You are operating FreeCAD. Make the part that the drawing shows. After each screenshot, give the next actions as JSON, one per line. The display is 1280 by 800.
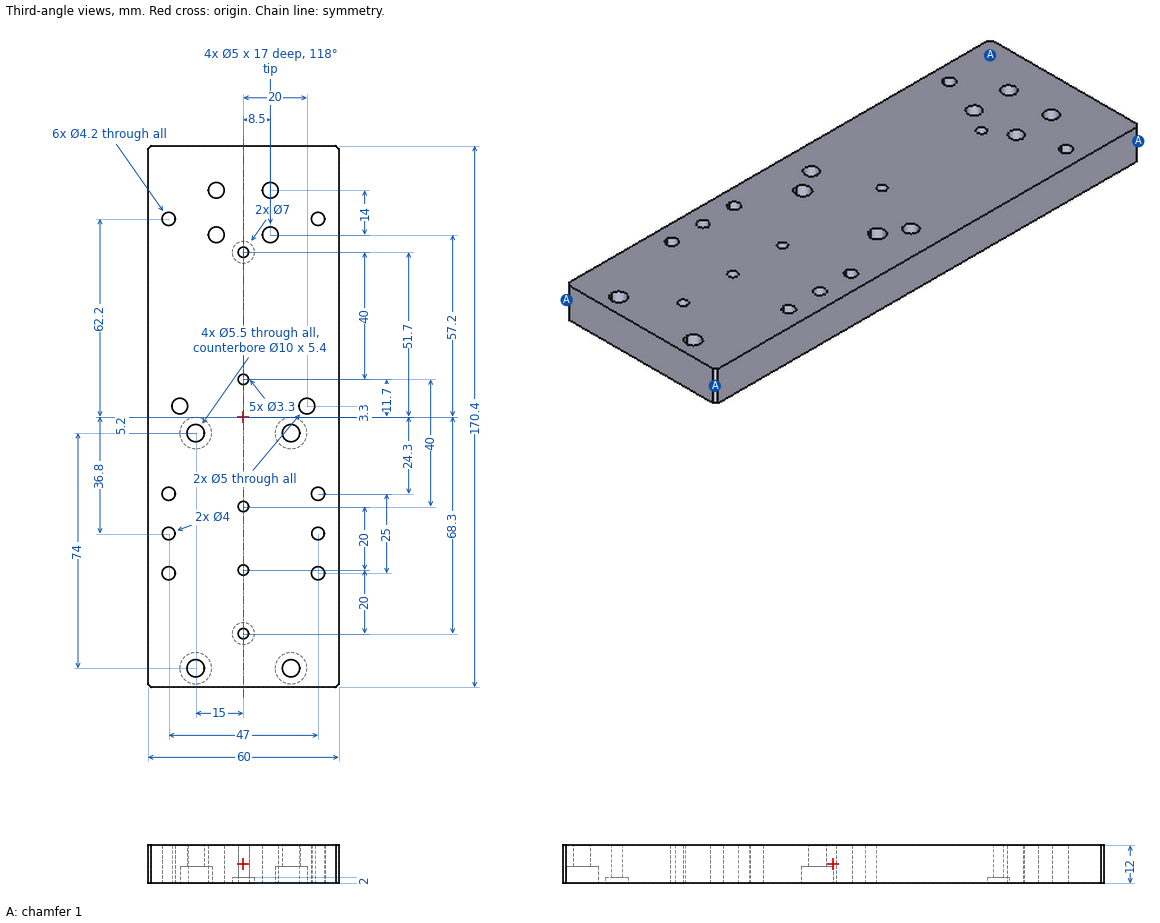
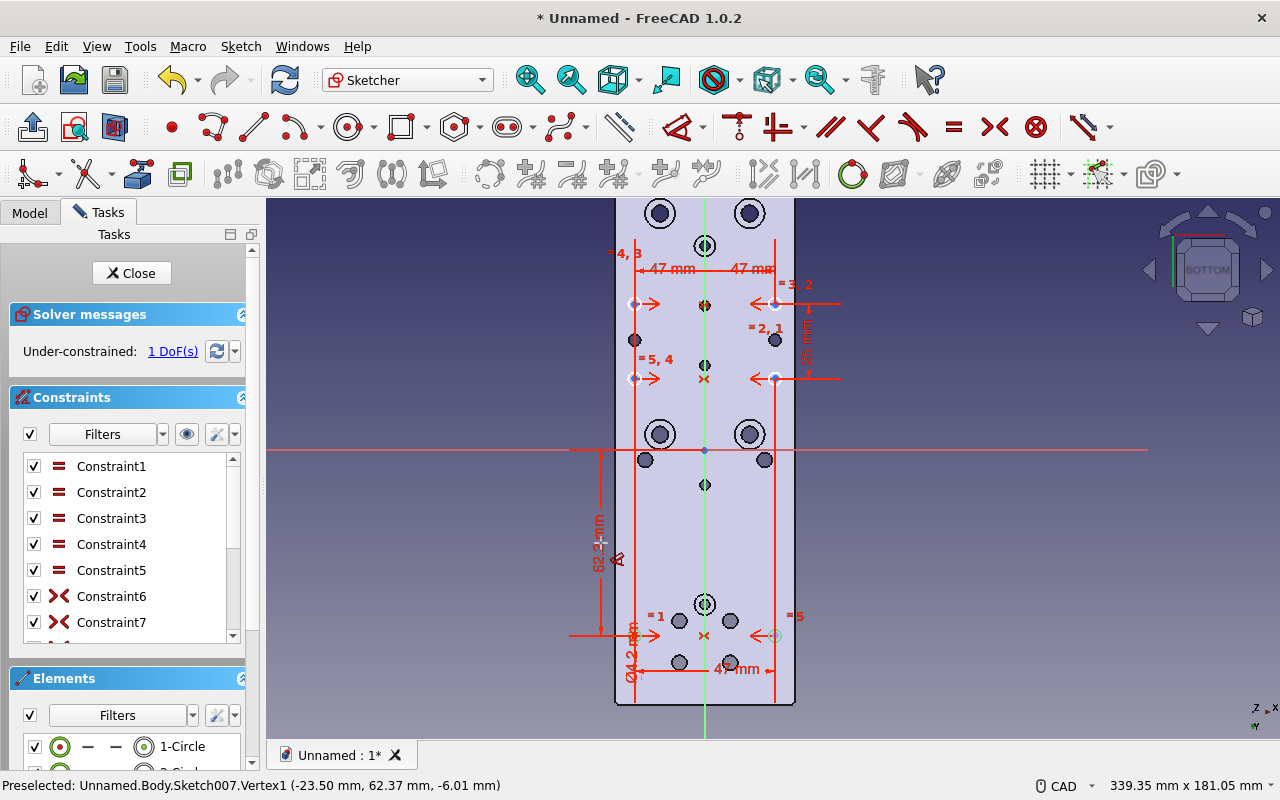
{"action": "left_click", "coordinate": [775, 379]}
{"action": "left_click", "coordinate": [809, 414]}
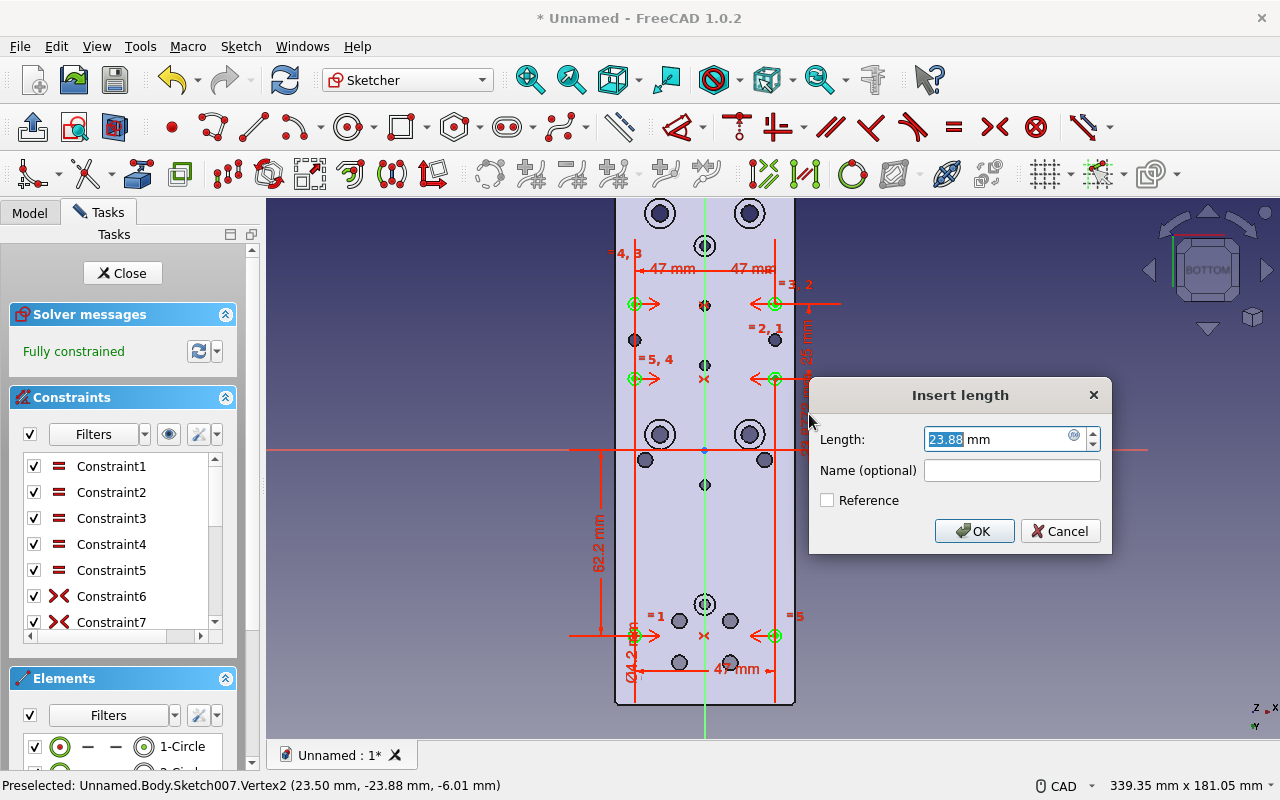
{"action": "type", "text": "24.3"}
{"action": "key", "text": "Return"}
{"action": "key", "text": "Escape"}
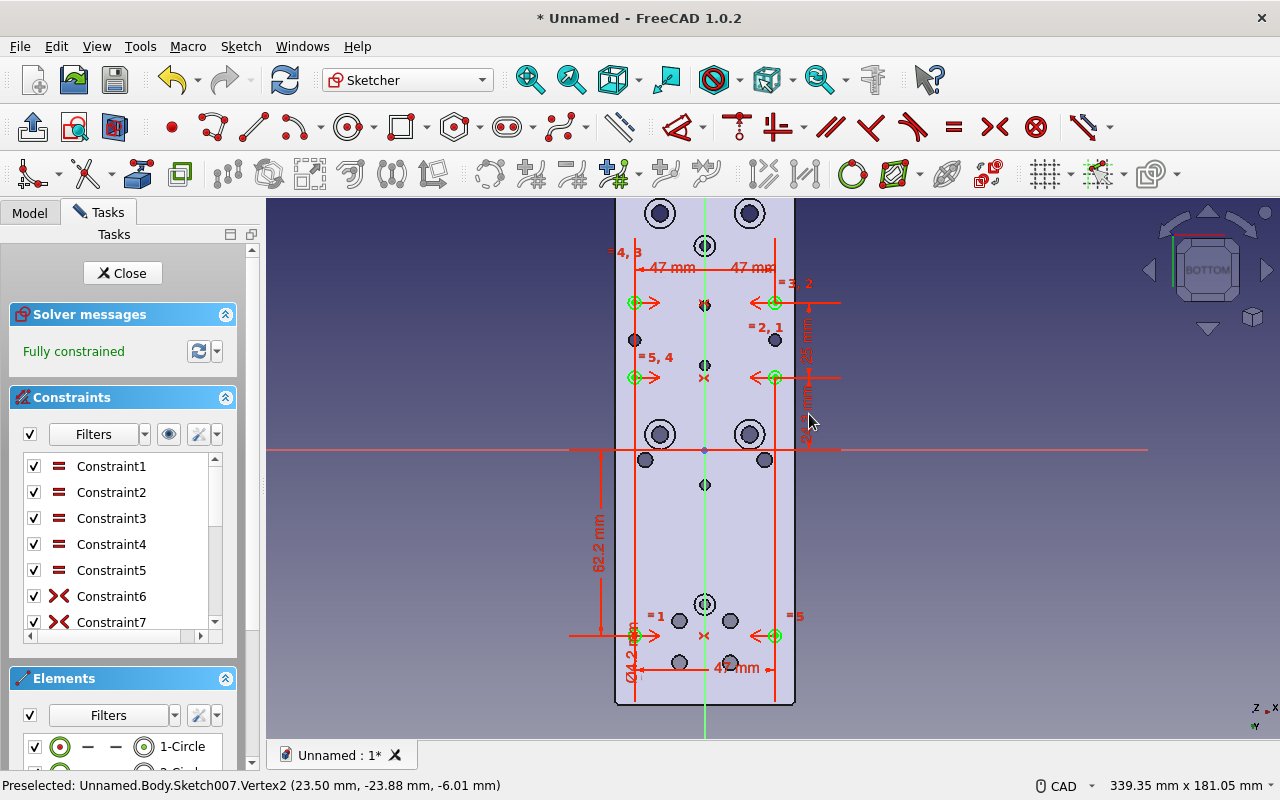
{"action": "left_click", "coordinate": [123, 273]}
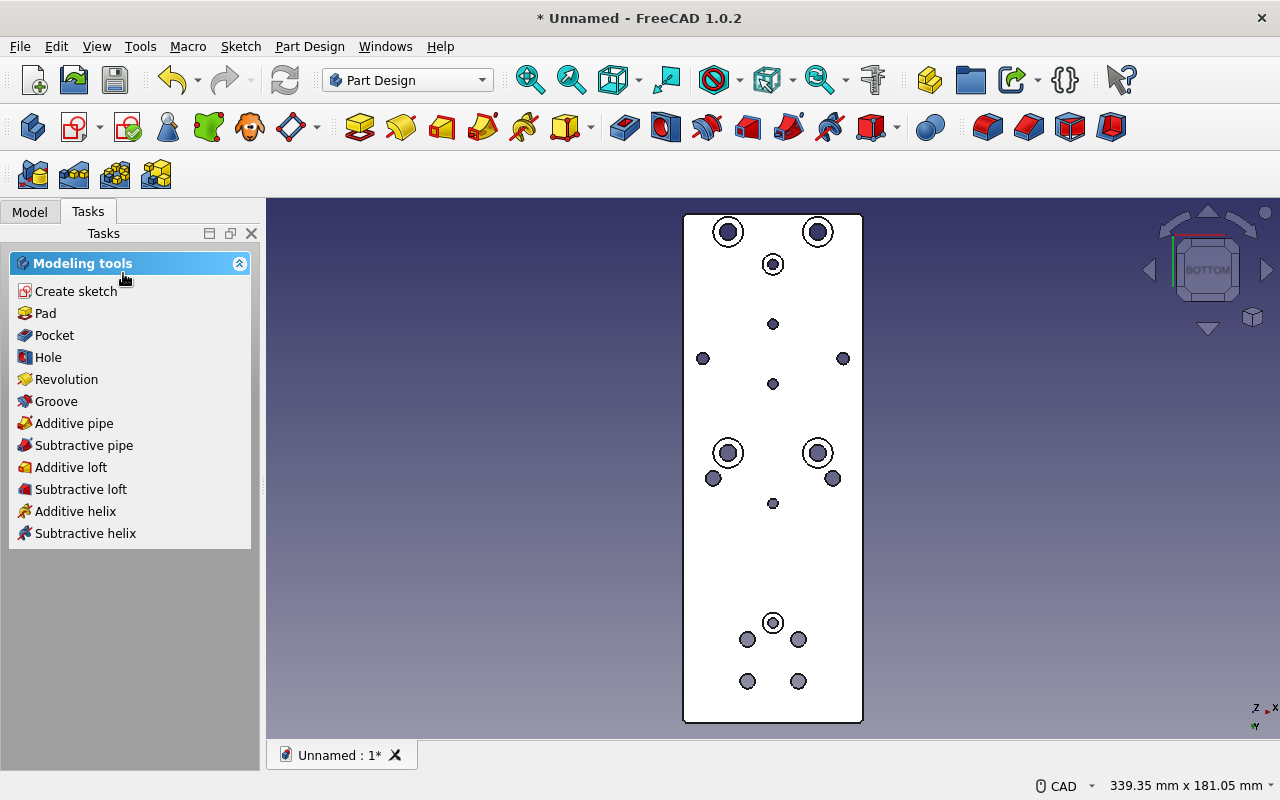
{"action": "left_click", "coordinate": [666, 128]}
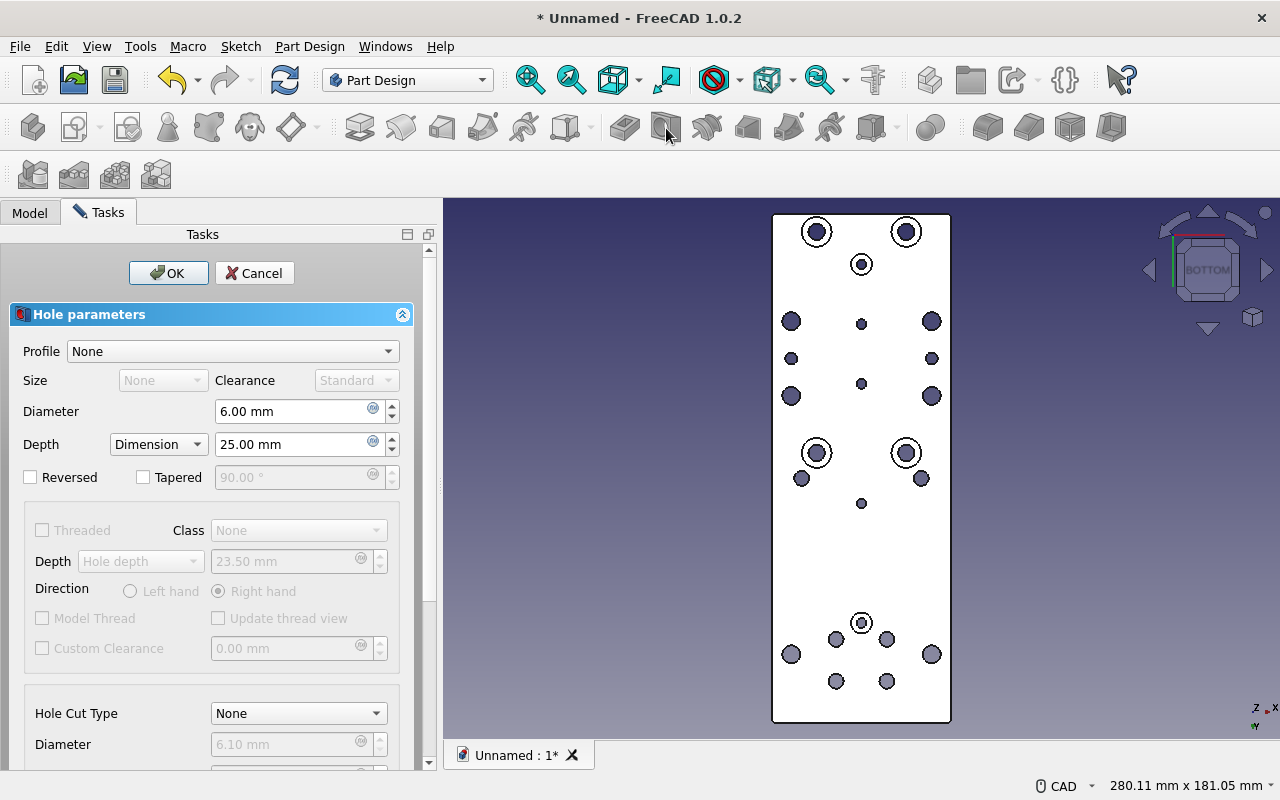
{"action": "triple_click", "coordinate": [300, 412]}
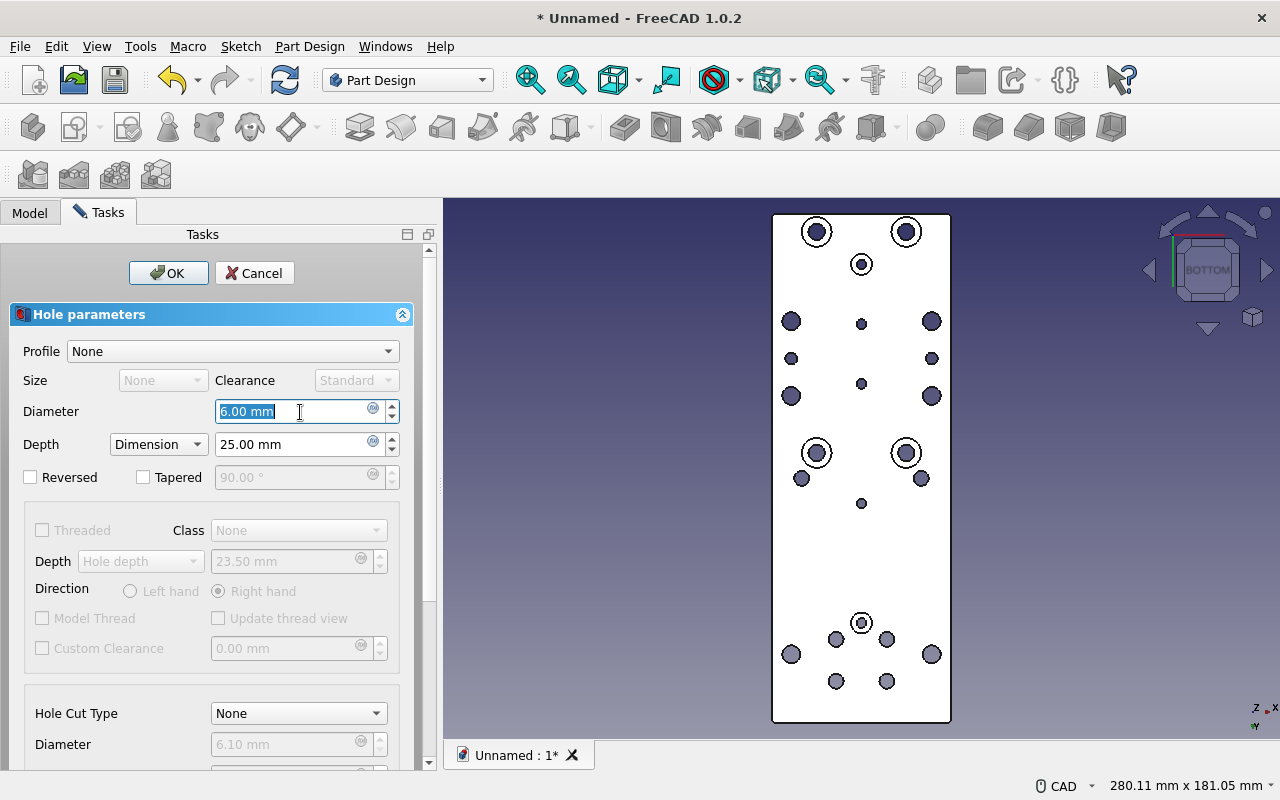
{"action": "type", "text": "4.2"}
{"action": "key", "text": "Tab"}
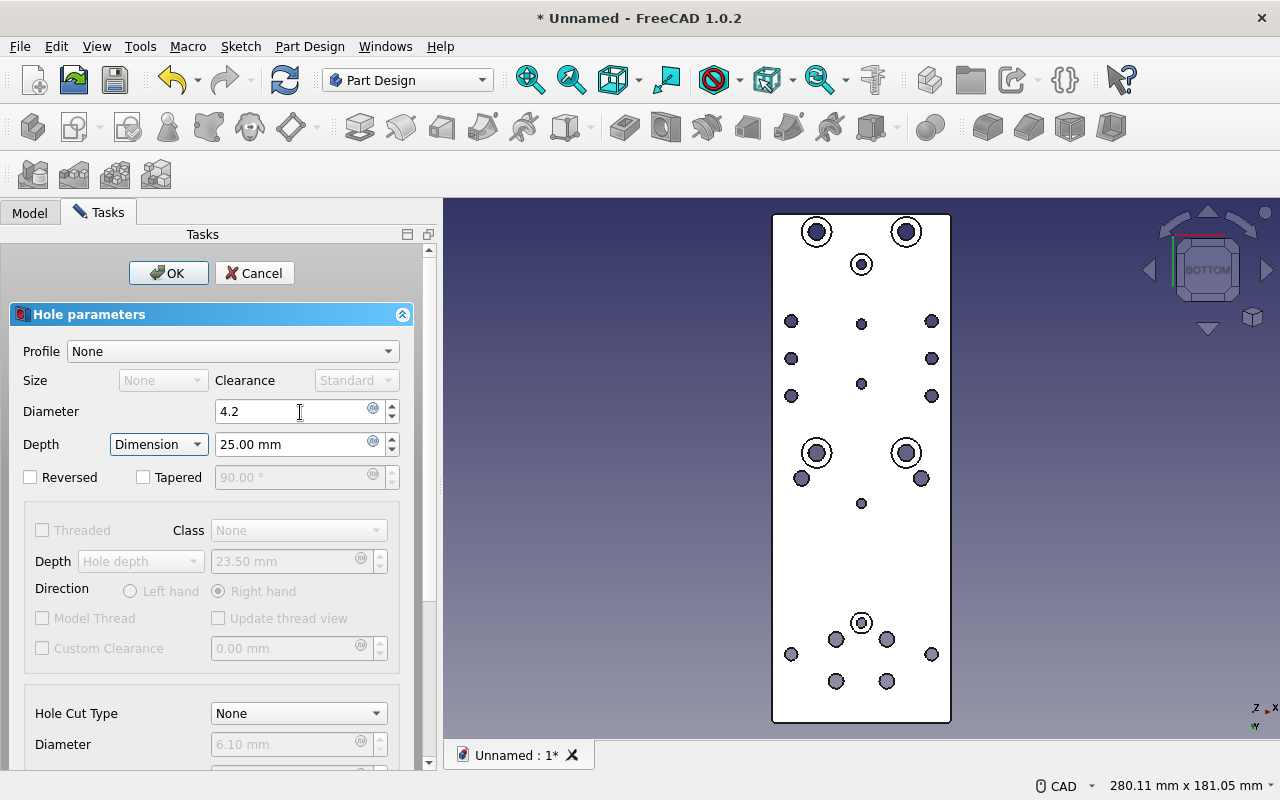
{"action": "left_click", "coordinate": [160, 444]}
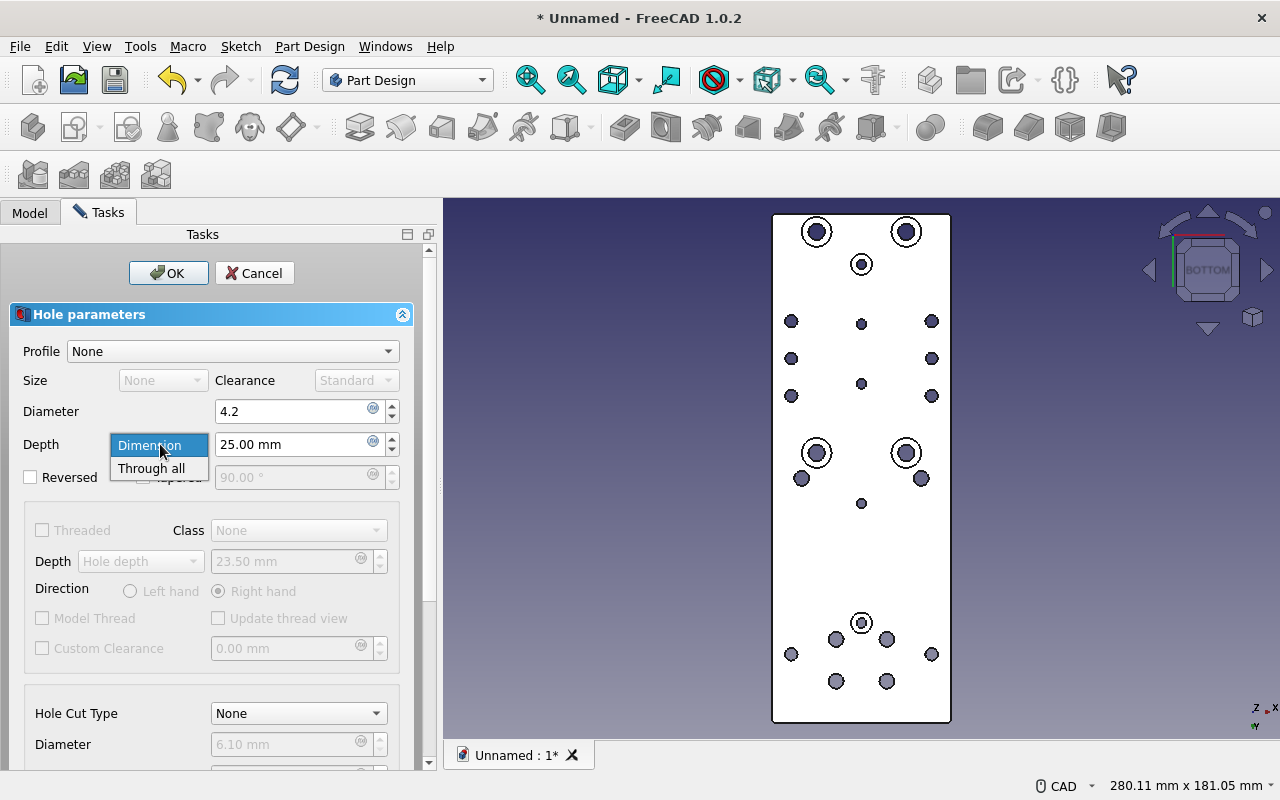
{"action": "left_click", "coordinate": [158, 468]}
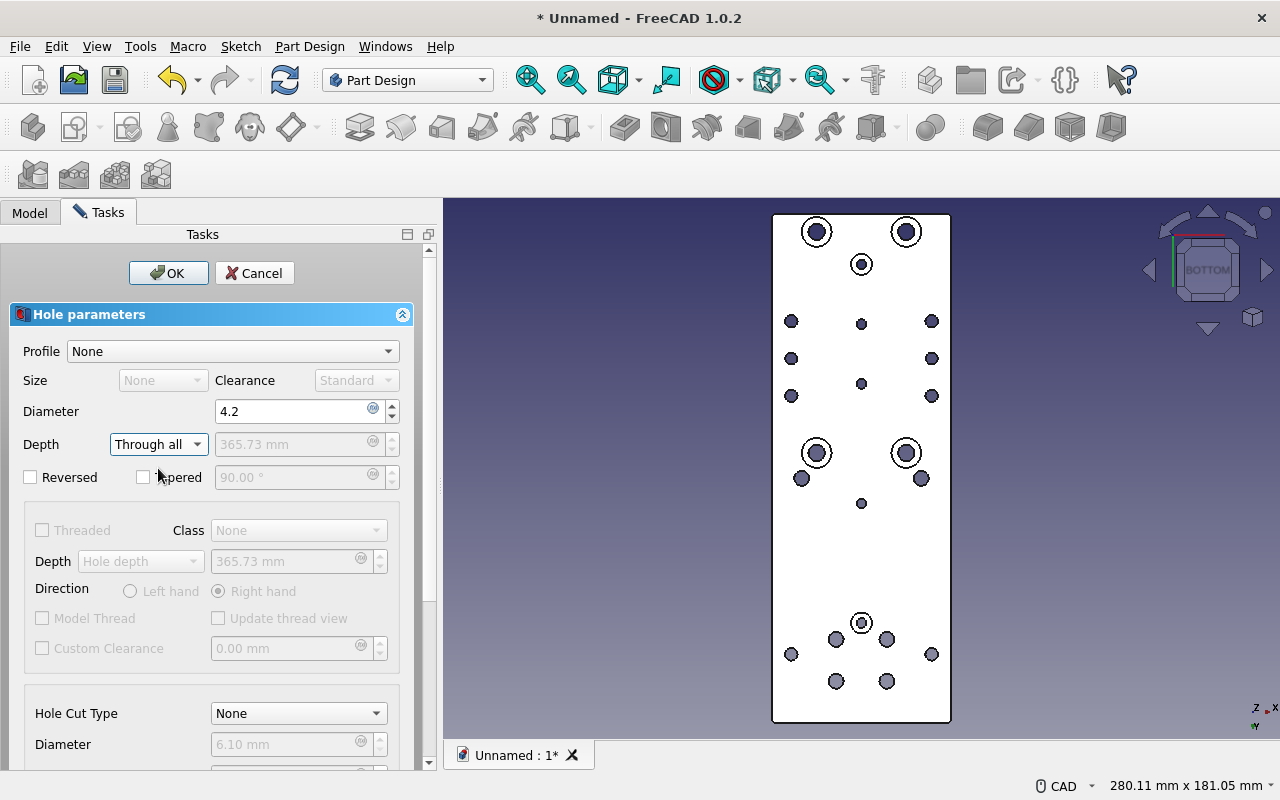
{"action": "left_click", "coordinate": [169, 273]}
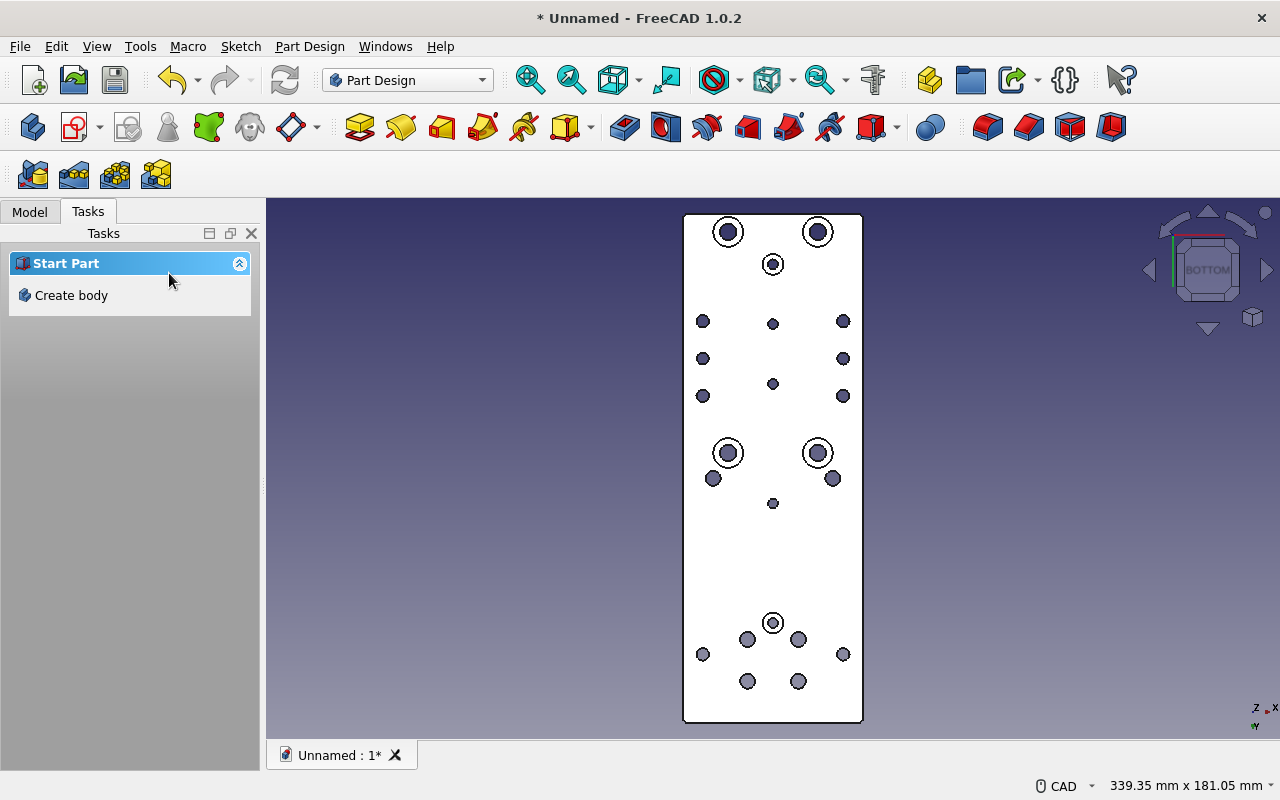
{"action": "key", "text": "0"}